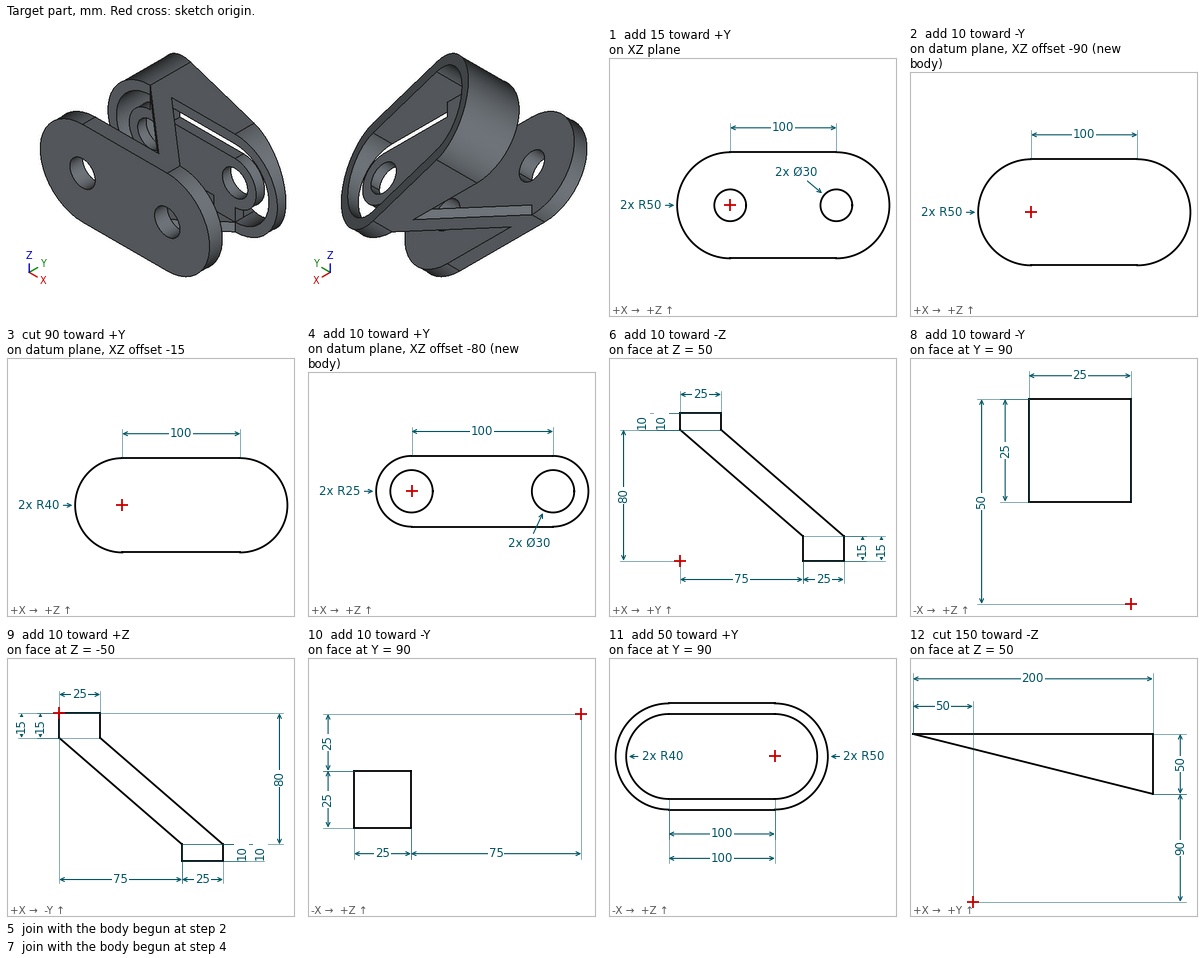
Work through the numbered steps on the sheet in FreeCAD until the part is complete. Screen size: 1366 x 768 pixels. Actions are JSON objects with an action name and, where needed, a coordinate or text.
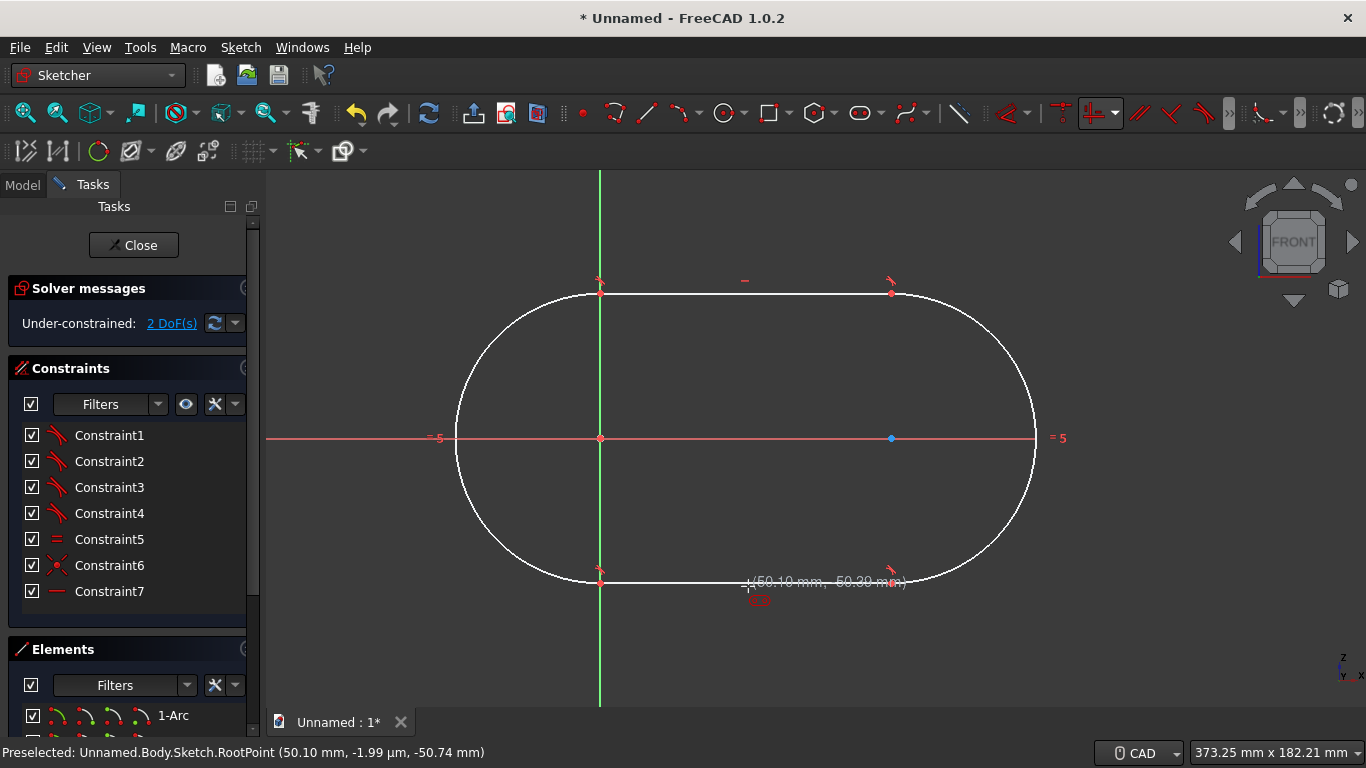
{"action": "left_click", "coordinate": [724, 114]}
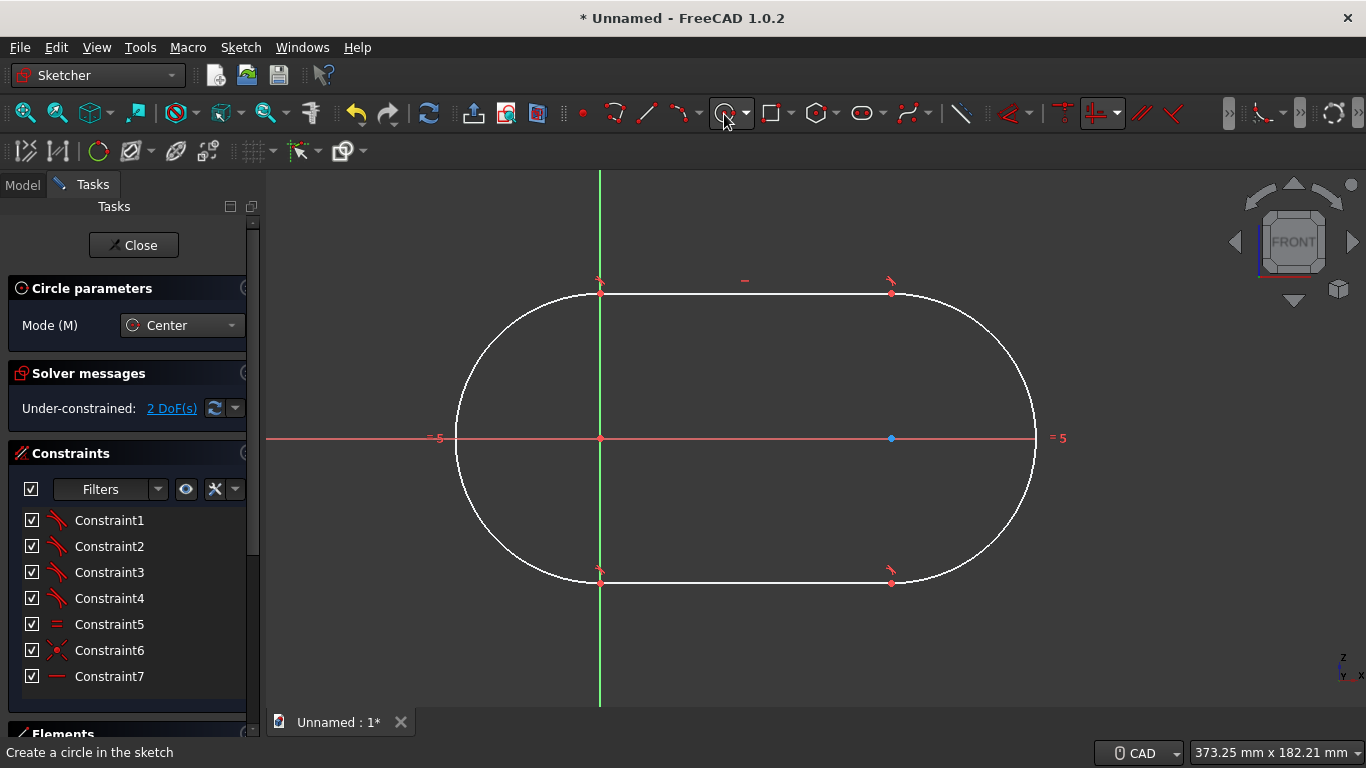
{"action": "left_click", "coordinate": [895, 430]}
{"action": "left_click", "coordinate": [926, 407]}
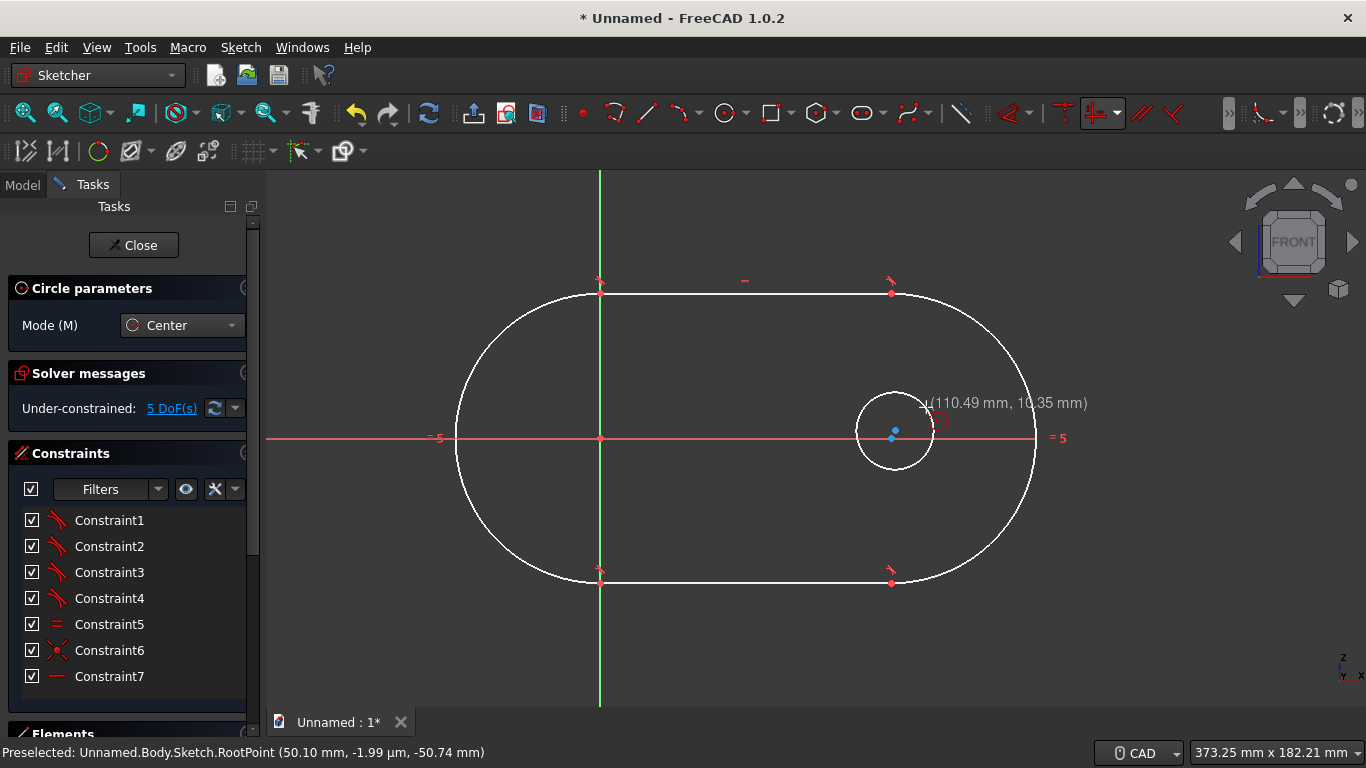
{"action": "left_click", "coordinate": [600, 438]}
{"action": "left_click", "coordinate": [632, 407]}
{"action": "key", "text": "Escape"}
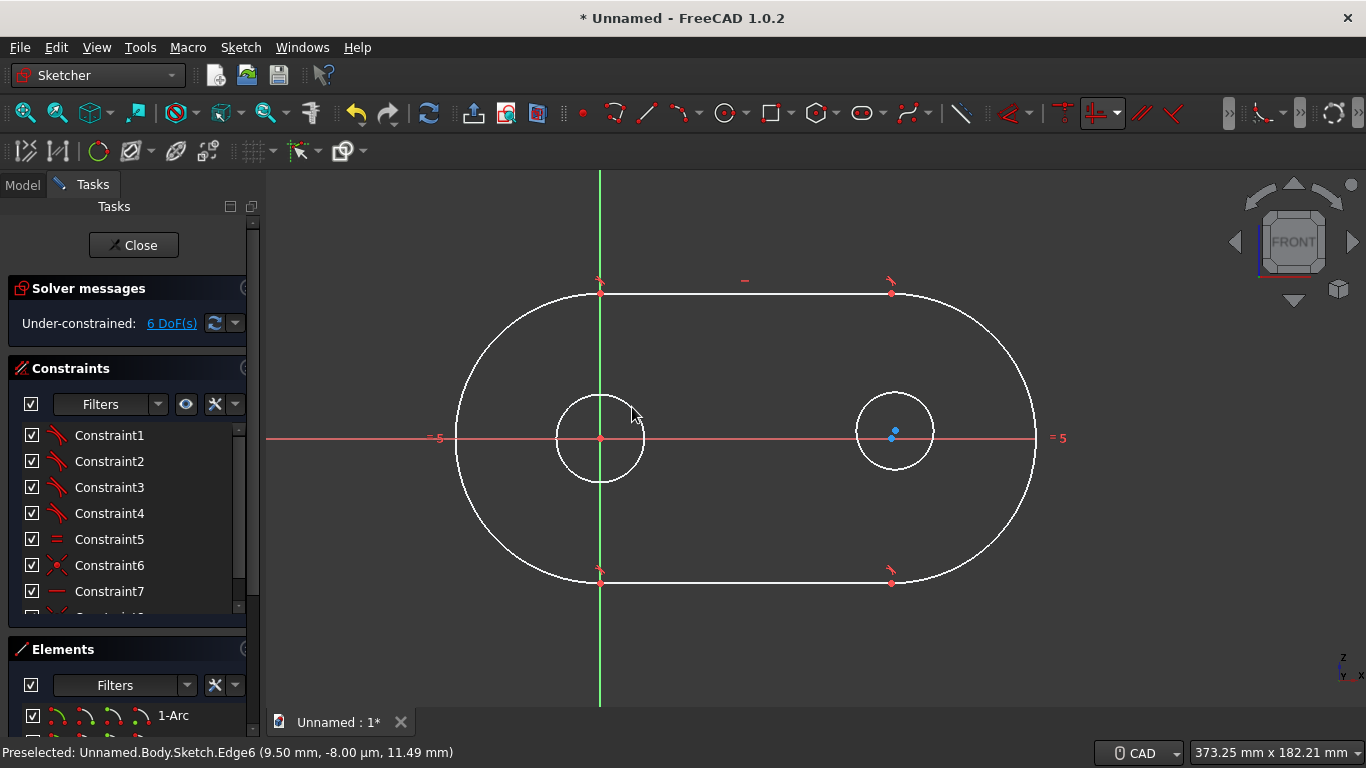
{"action": "left_click", "coordinate": [922, 404]}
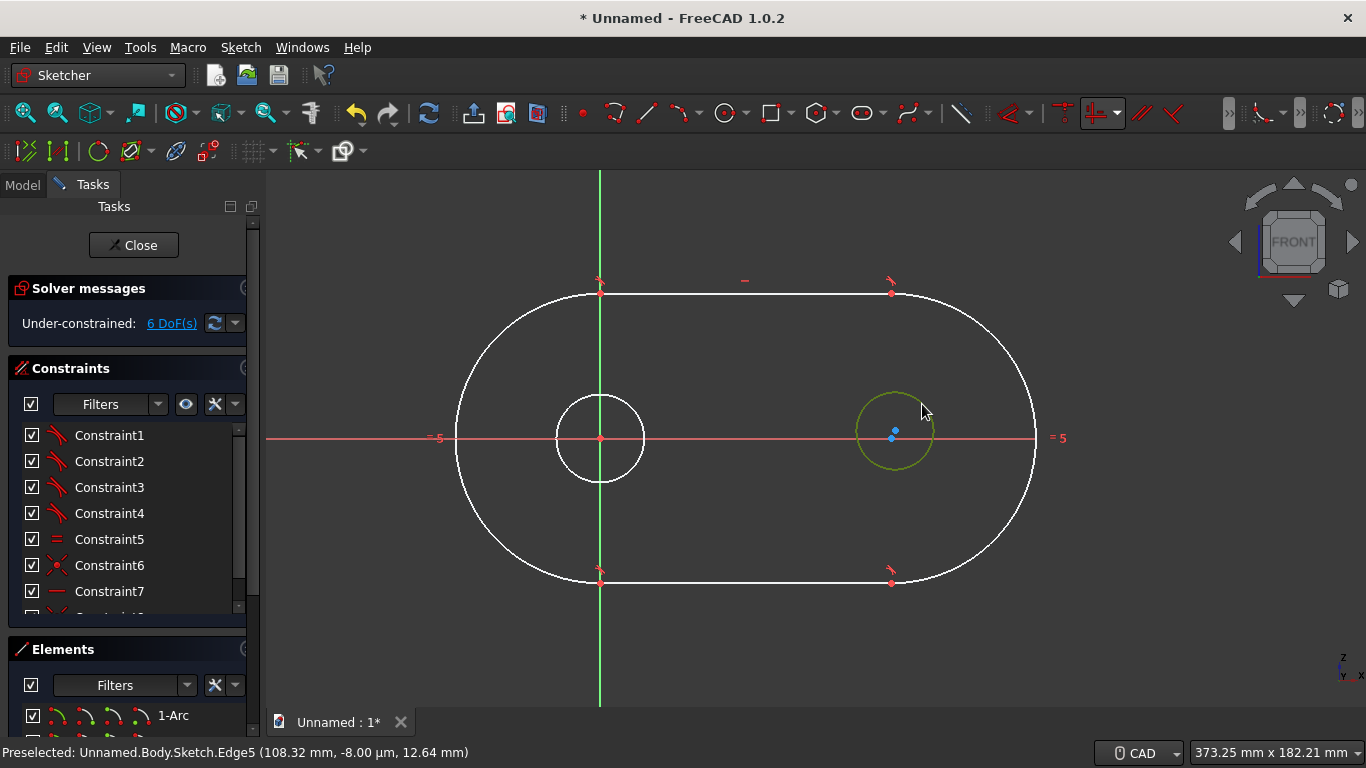
{"action": "left_click", "coordinate": [1008, 524]}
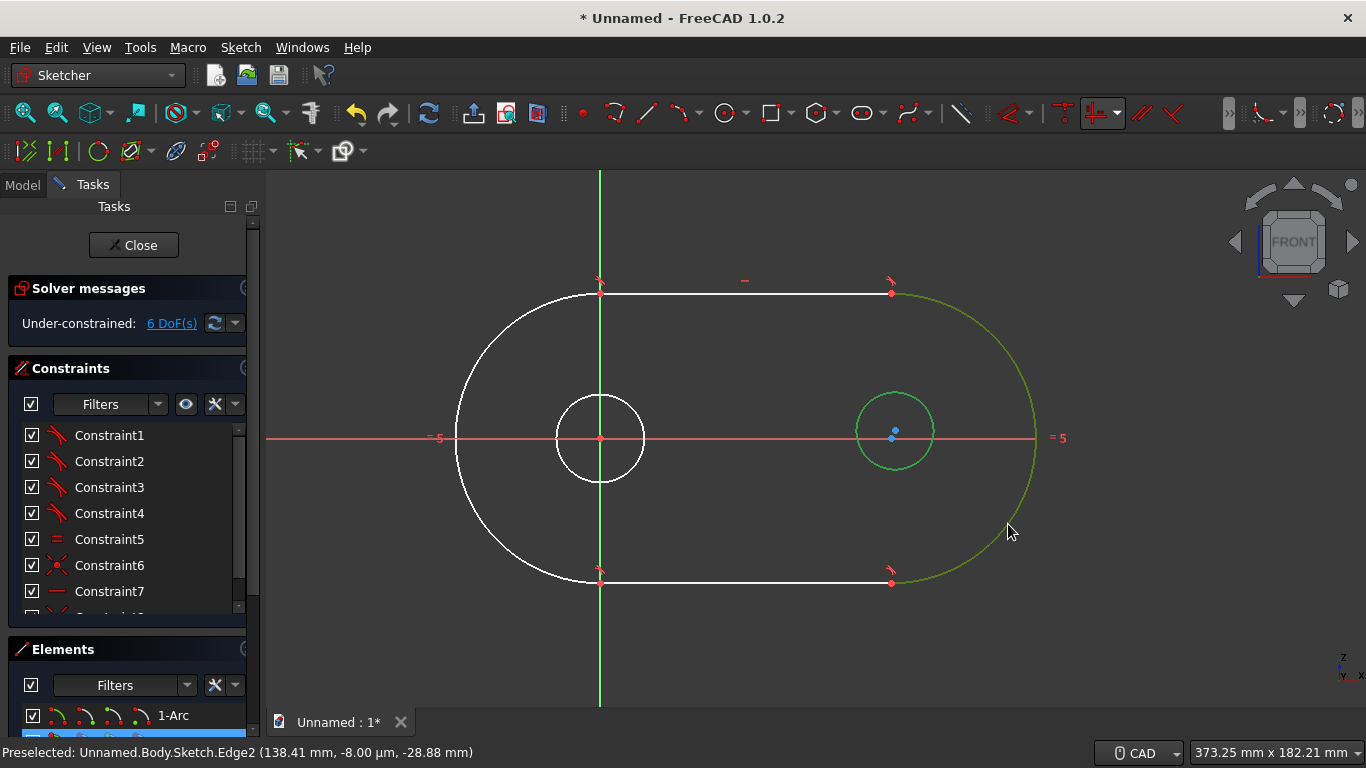
{"action": "left_click", "coordinate": [1064, 114]}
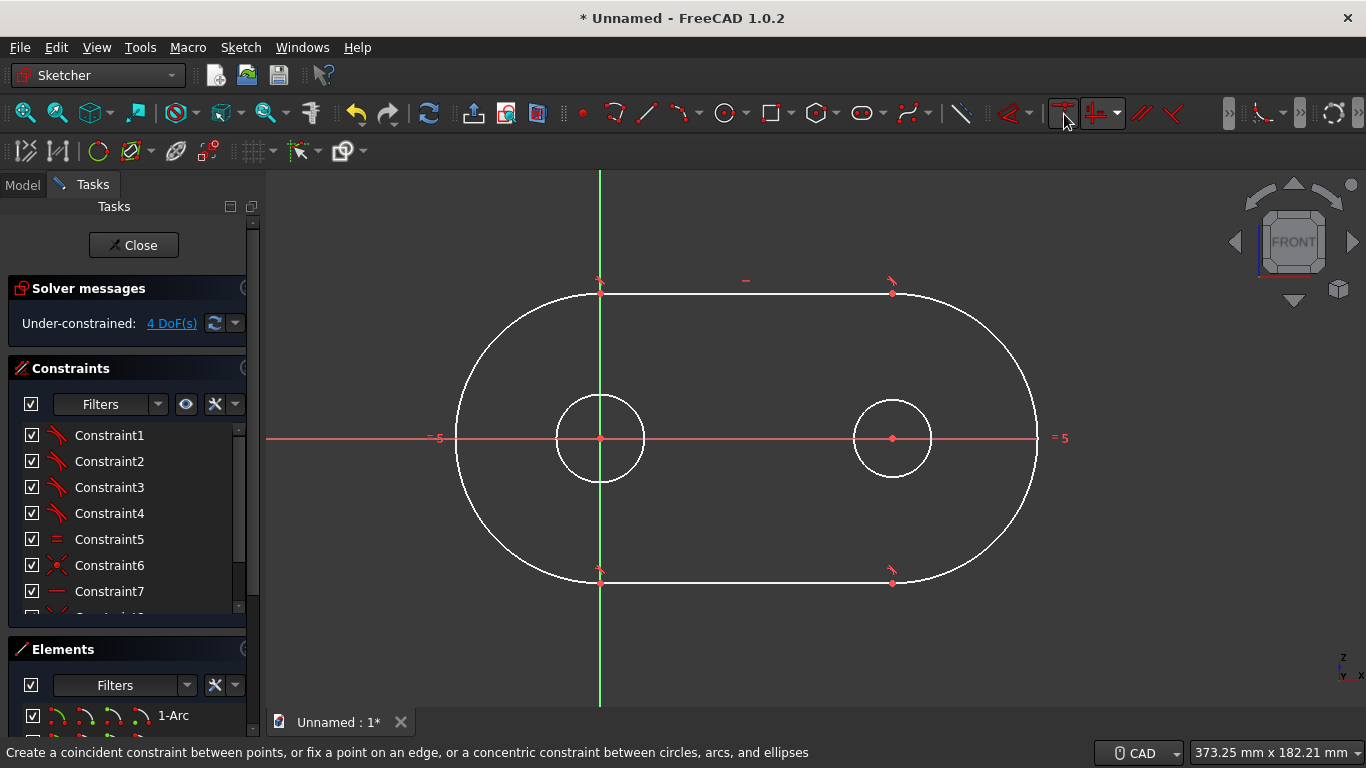
{"action": "left_click", "coordinate": [920, 411]}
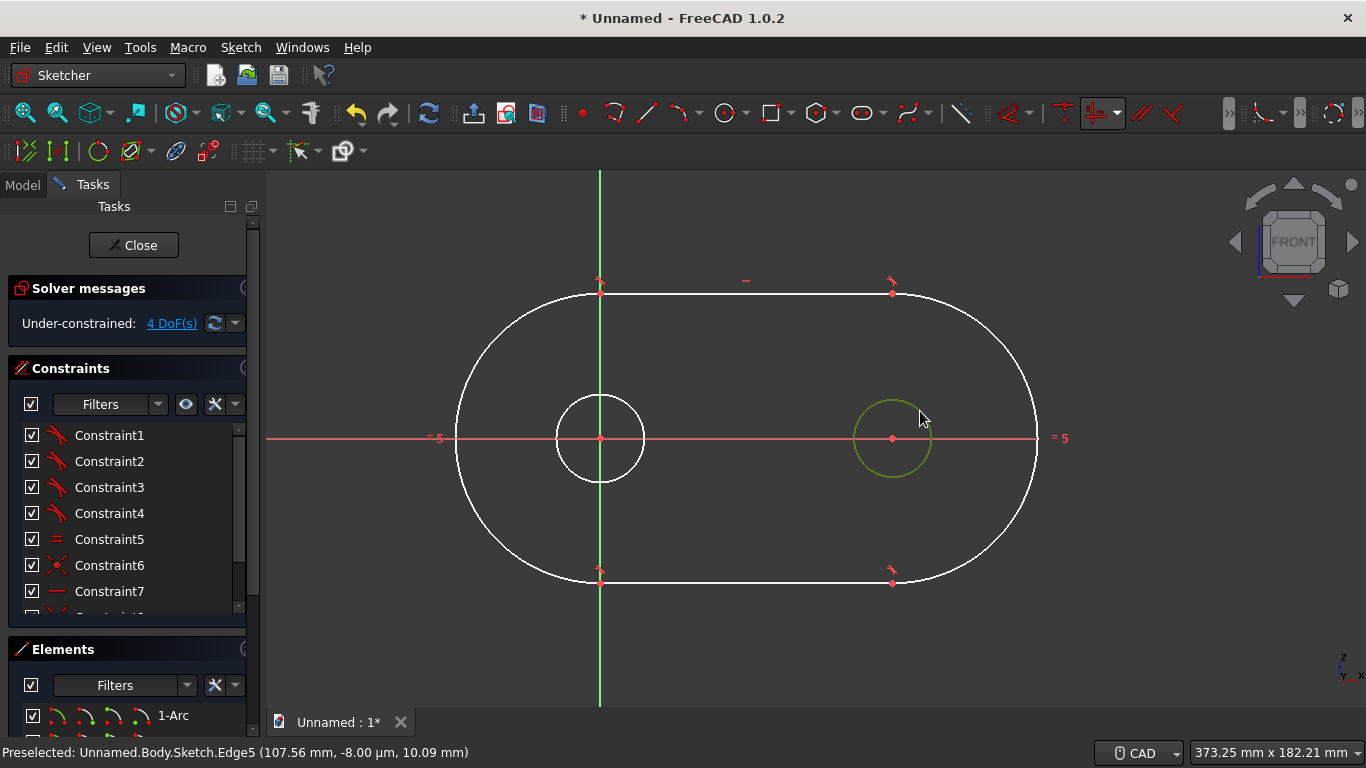
{"action": "left_click", "coordinate": [631, 407]}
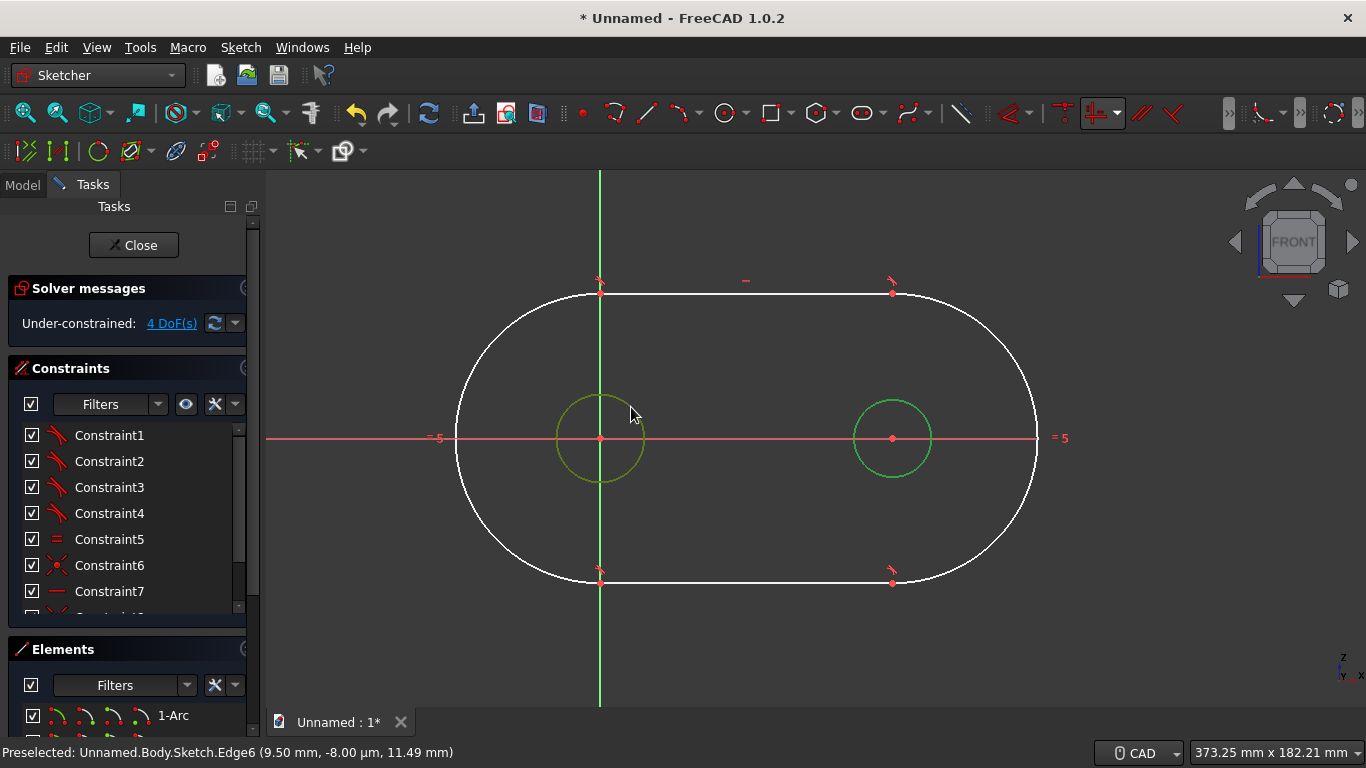
{"action": "key", "text": "e"}